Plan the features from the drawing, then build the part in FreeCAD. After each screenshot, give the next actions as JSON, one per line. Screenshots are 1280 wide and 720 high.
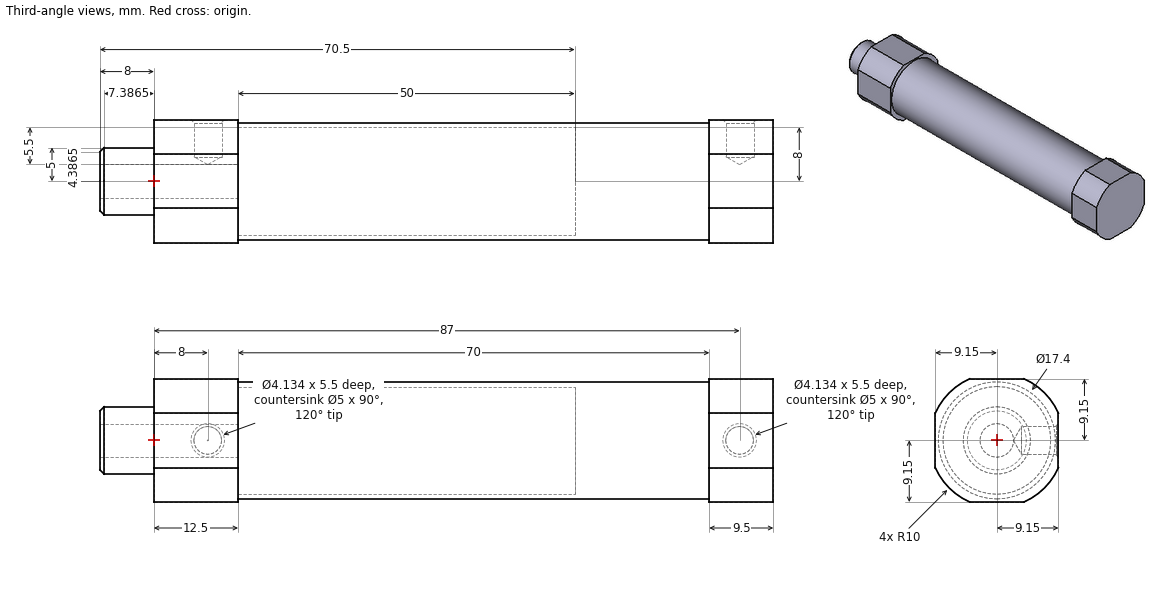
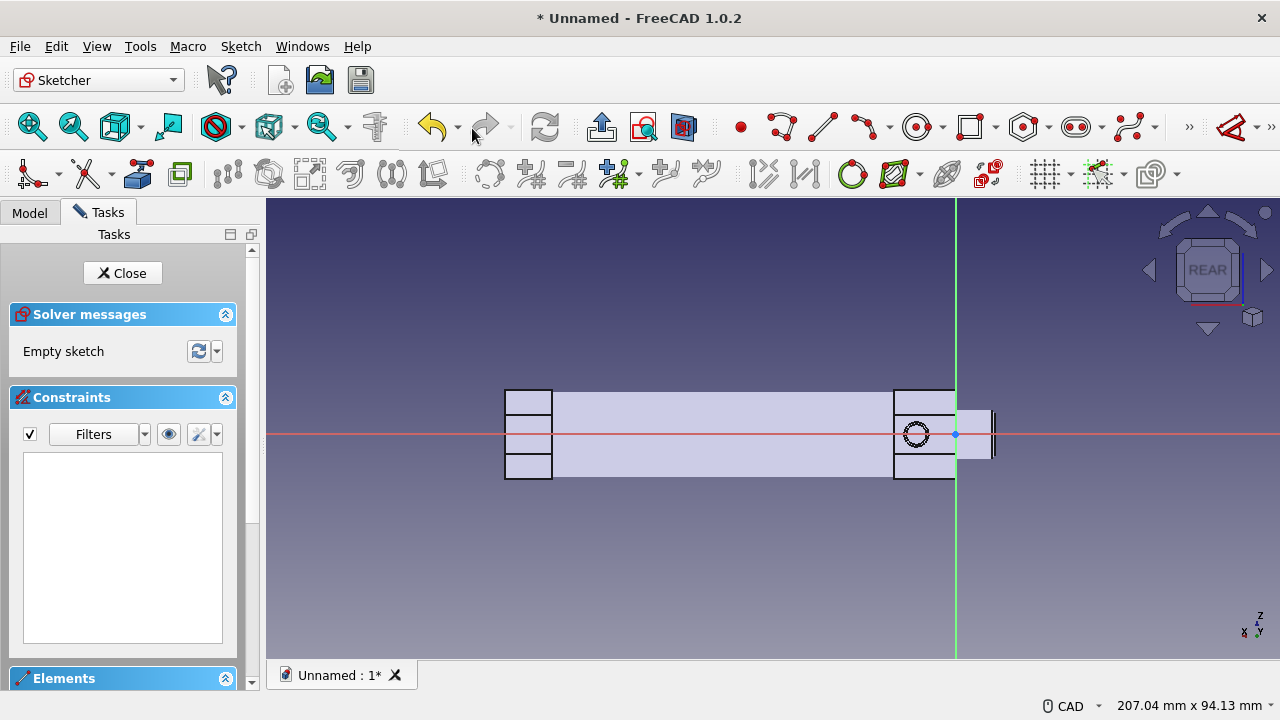
{"action": "scroll", "coordinate": [515, 435], "scroll_direction": "up", "scroll_amount": 13}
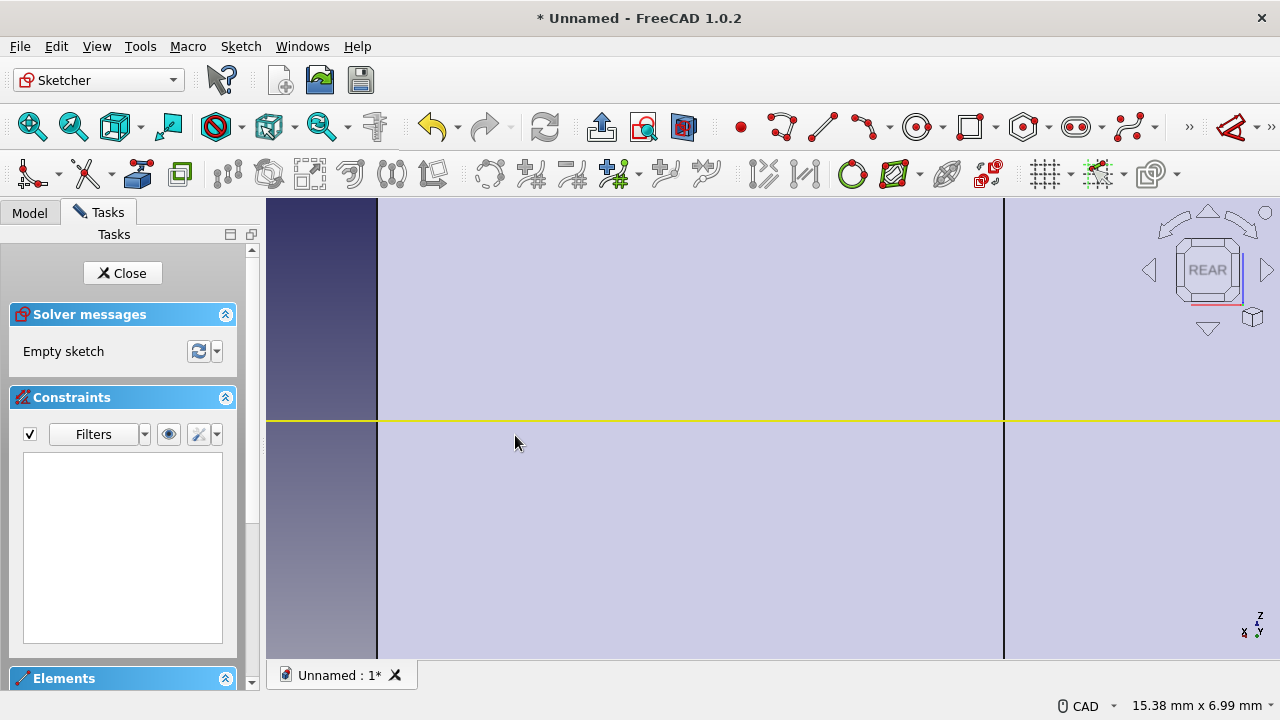
{"action": "left_click", "coordinate": [916, 128]}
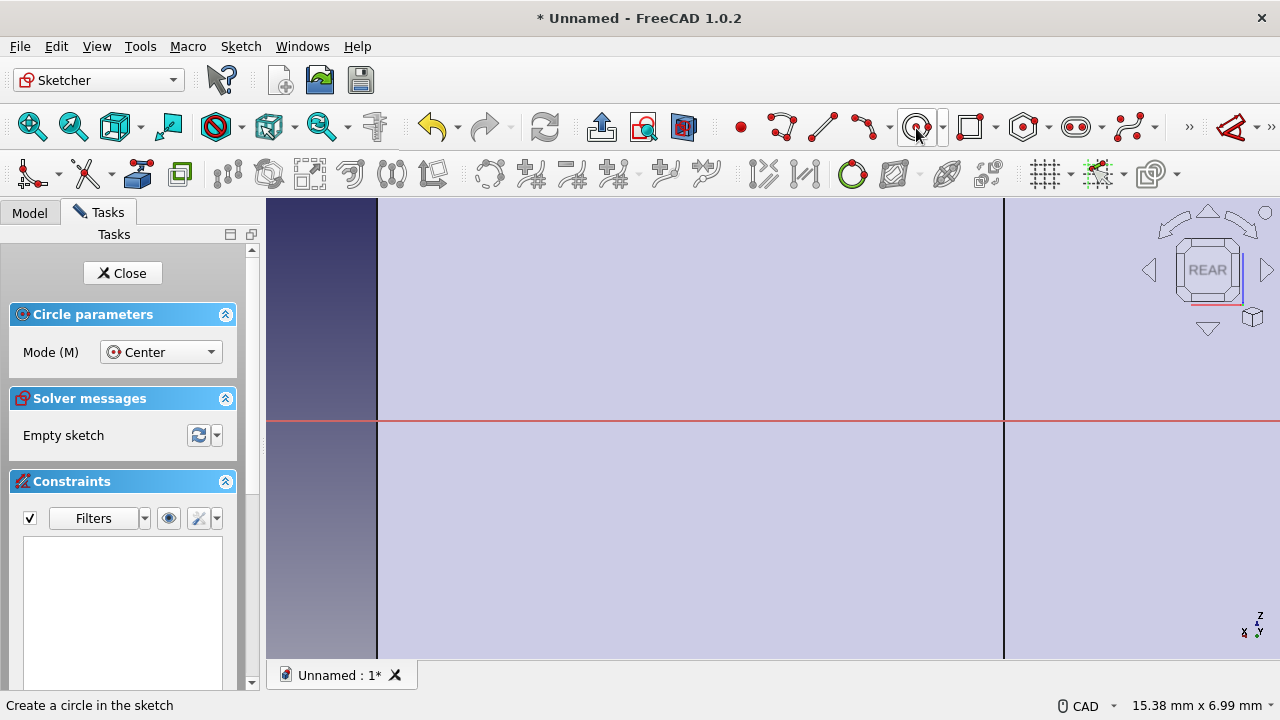
{"action": "left_click", "coordinate": [707, 421]}
{"action": "left_click", "coordinate": [803, 325]}
{"action": "key", "text": "Escape"}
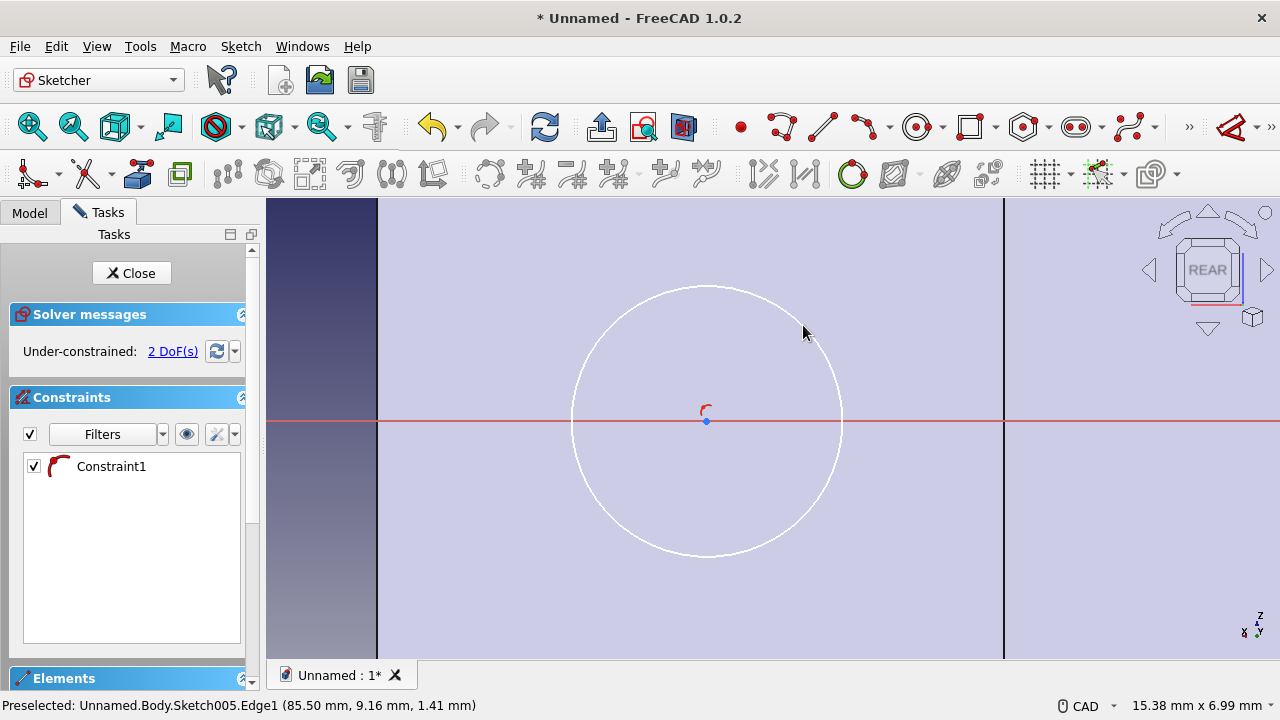
{"action": "key", "text": "d"}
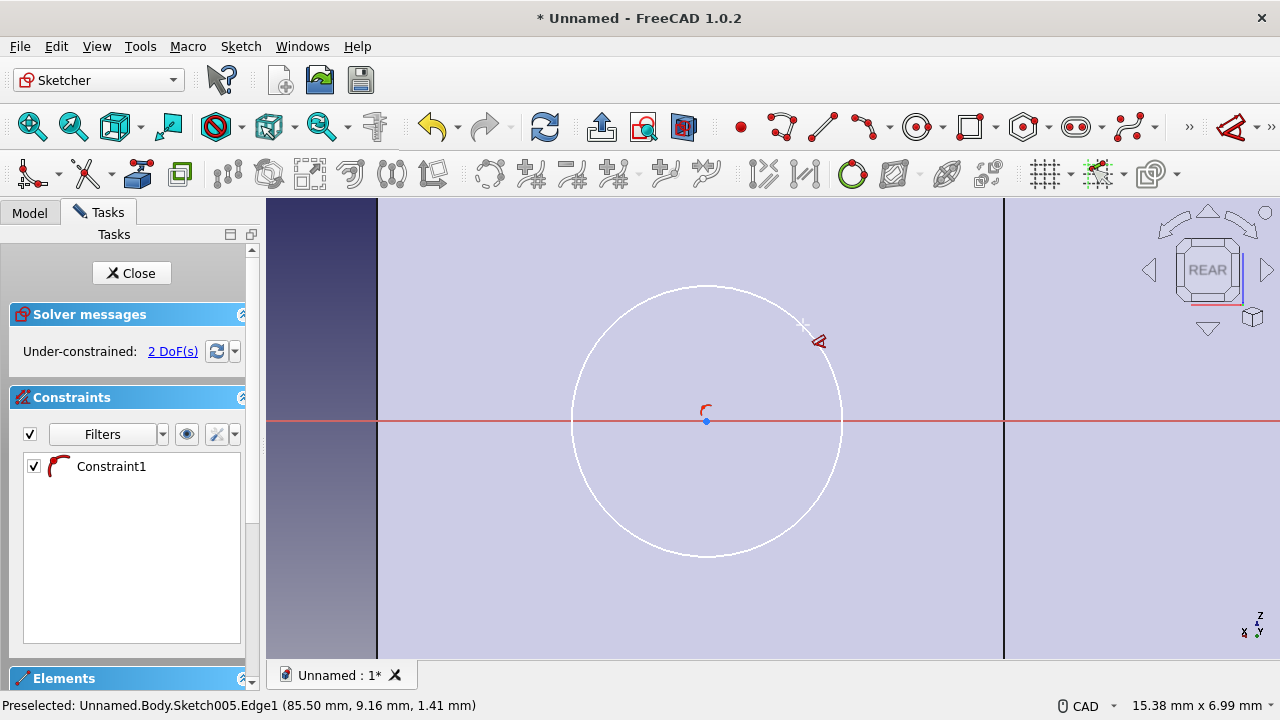
{"action": "left_click", "coordinate": [802, 325]}
{"action": "left_click", "coordinate": [824, 302]}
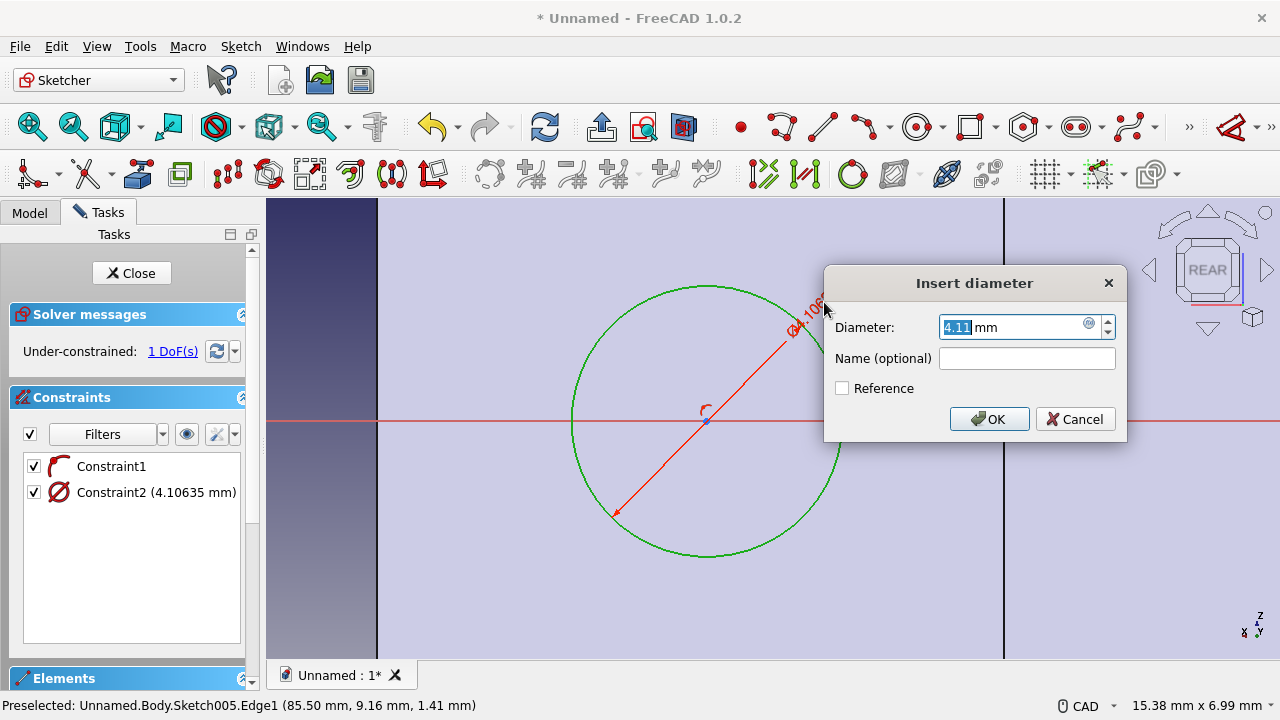
{"action": "type", "text": "4.134"}
{"action": "key", "text": "Return"}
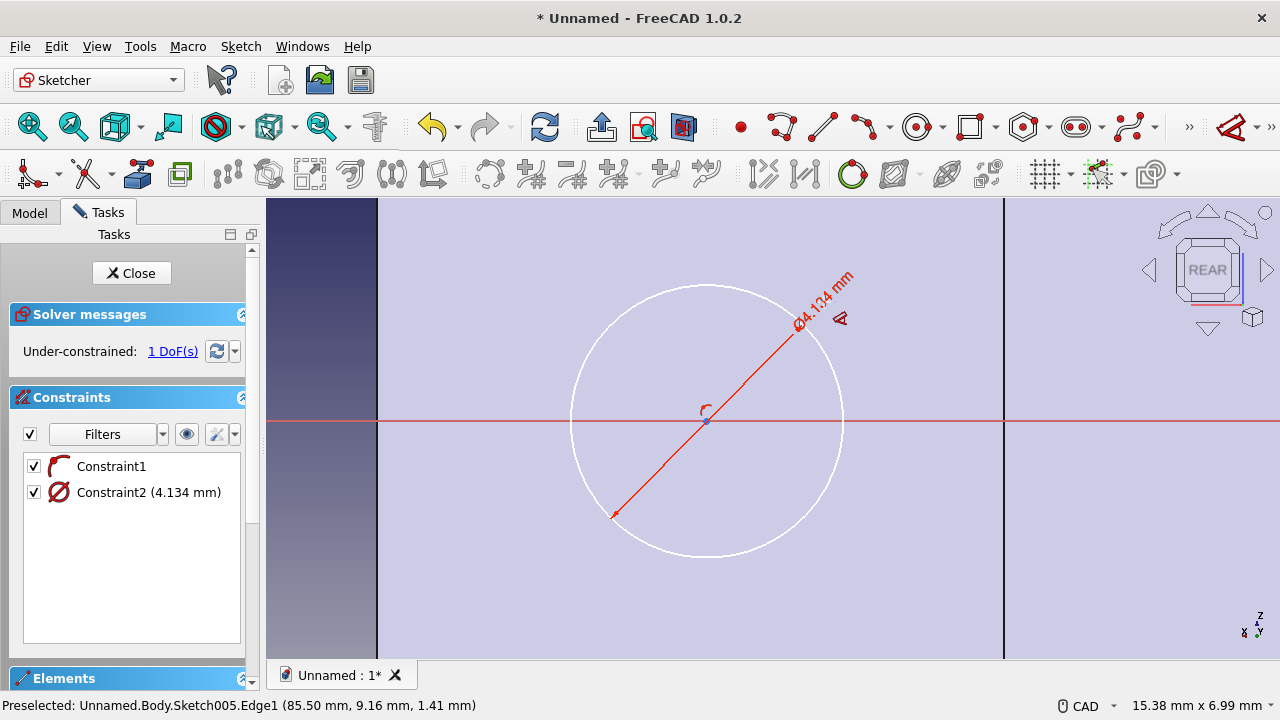
{"action": "left_click", "coordinate": [707, 421]}
{"action": "left_click", "coordinate": [911, 455]}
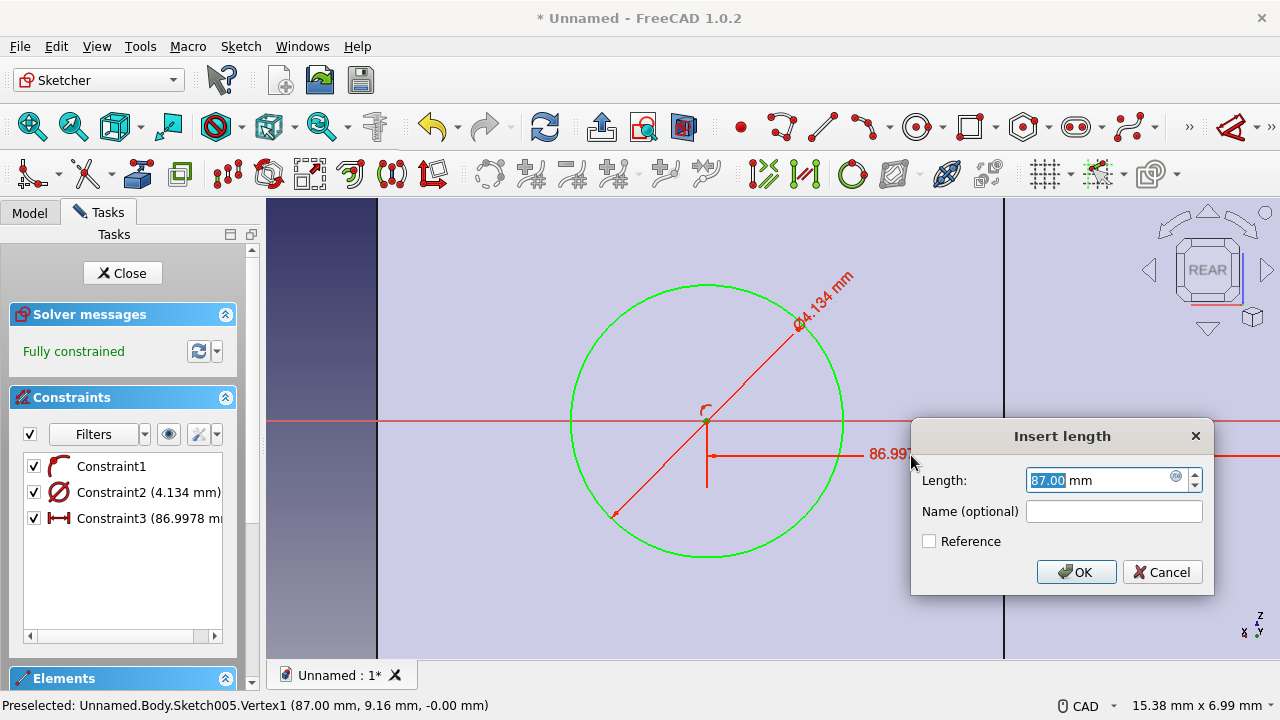
{"action": "type", "text": "87"}
{"action": "key", "text": "Return"}
{"action": "key", "text": "Escape"}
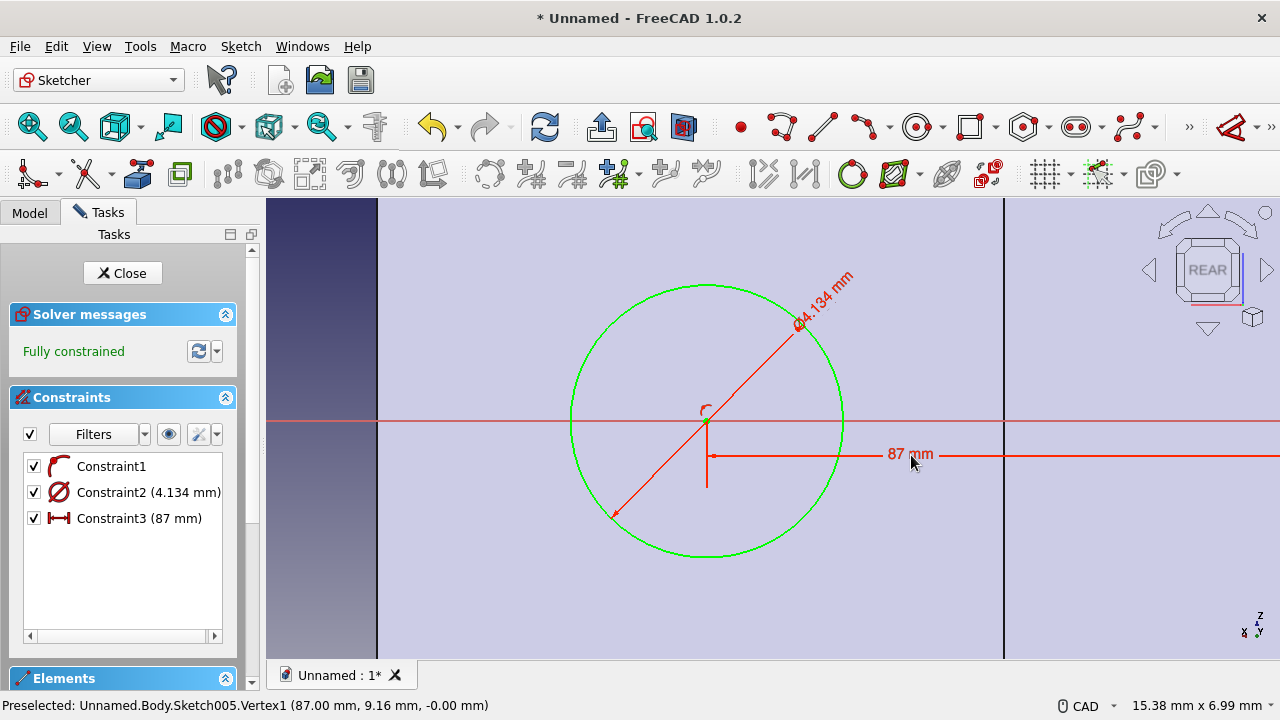
{"action": "left_click", "coordinate": [123, 273]}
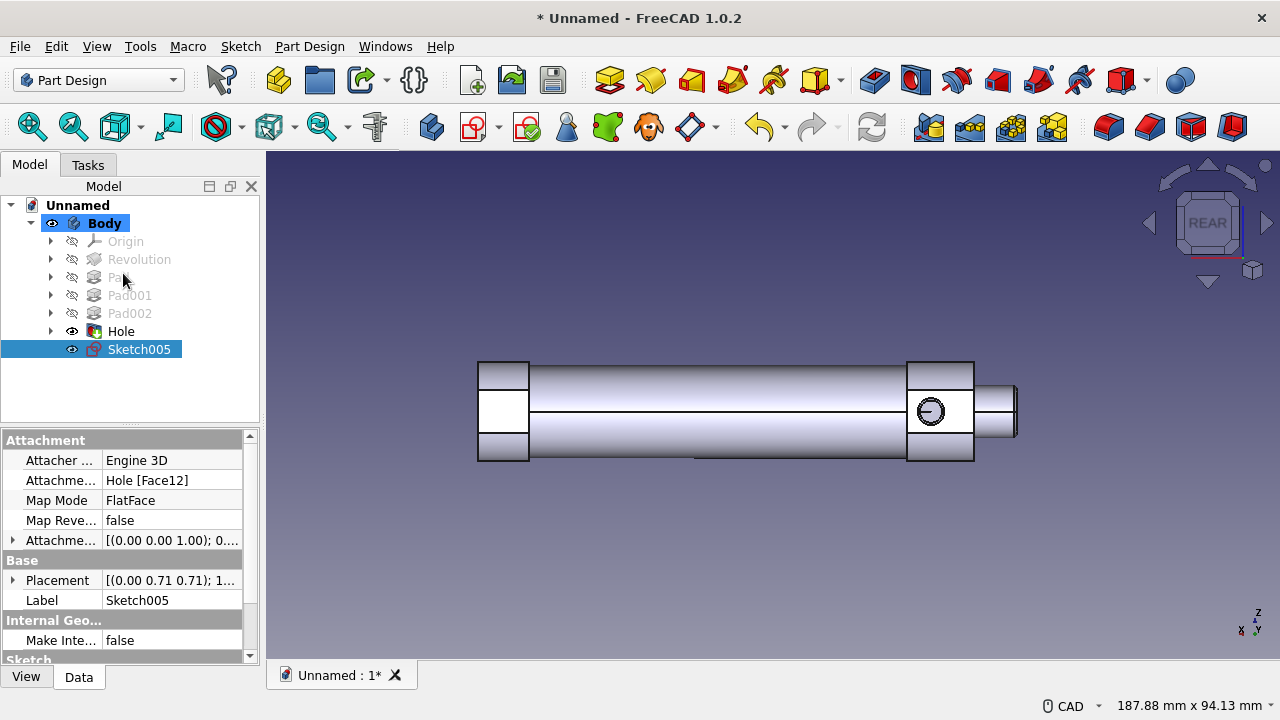
{"action": "left_click", "coordinate": [916, 80]}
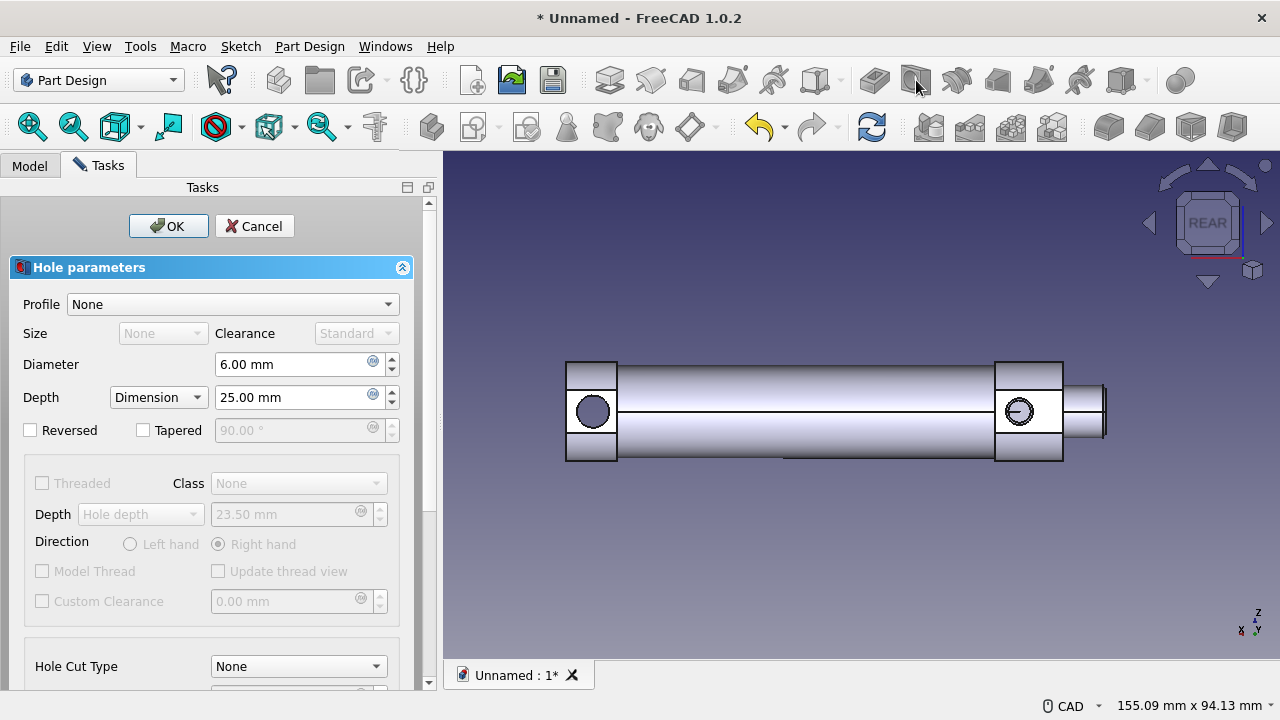
{"action": "triple_click", "coordinate": [300, 364]}